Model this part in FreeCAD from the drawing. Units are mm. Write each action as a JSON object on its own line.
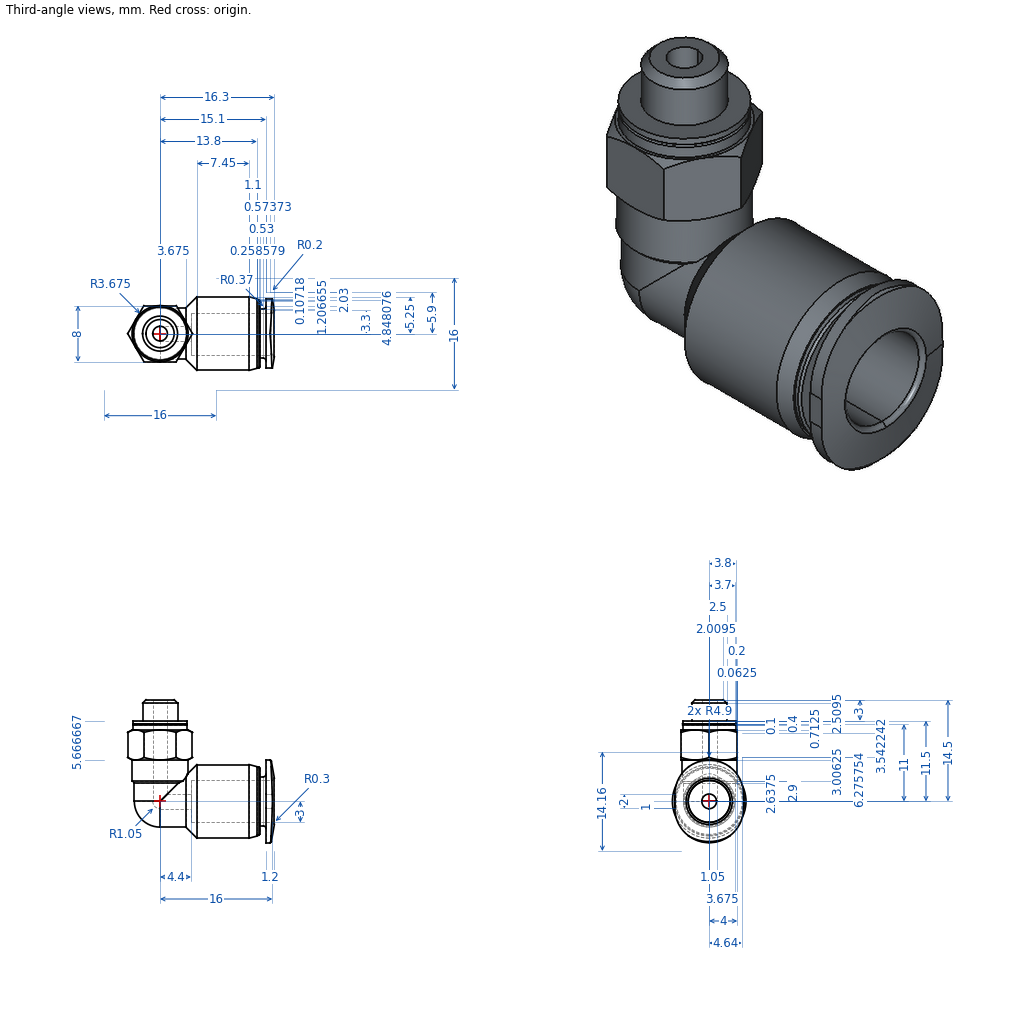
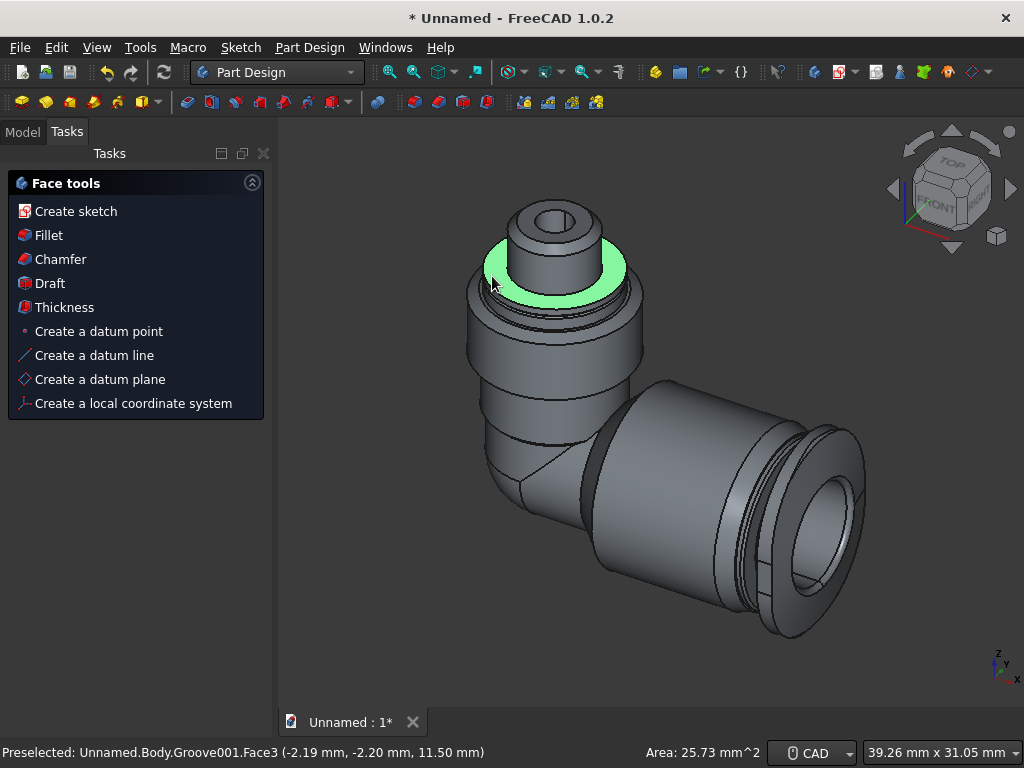
{"action": "left_click", "coordinate": [840, 72]}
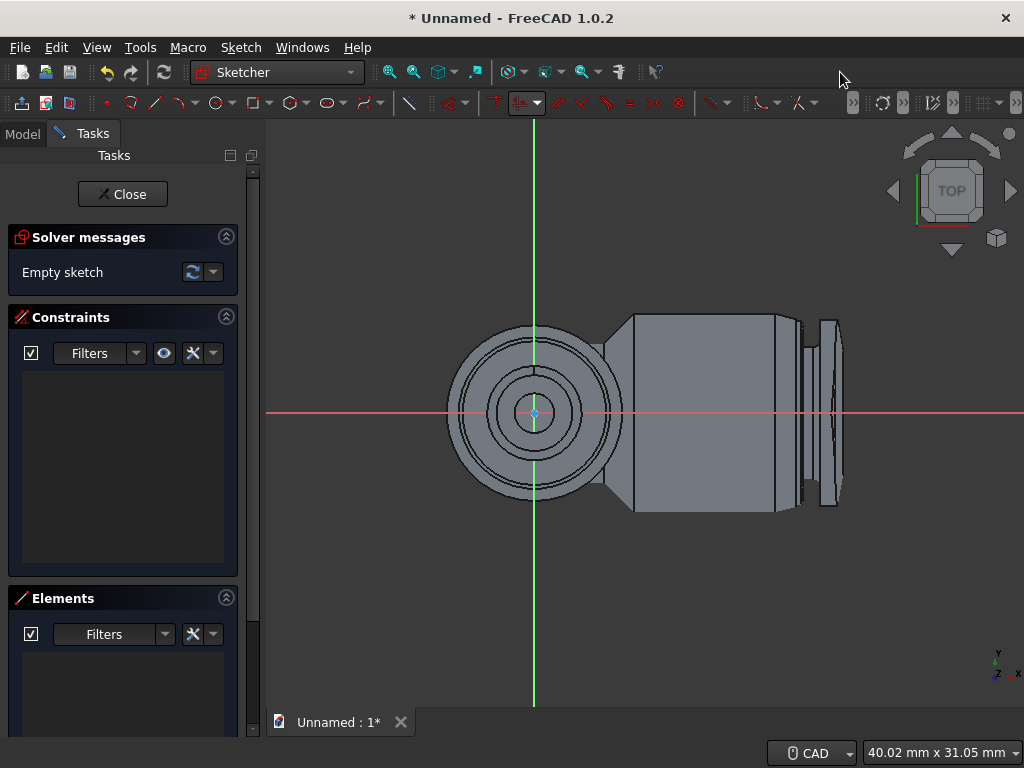
{"action": "left_click", "coordinate": [70, 104]}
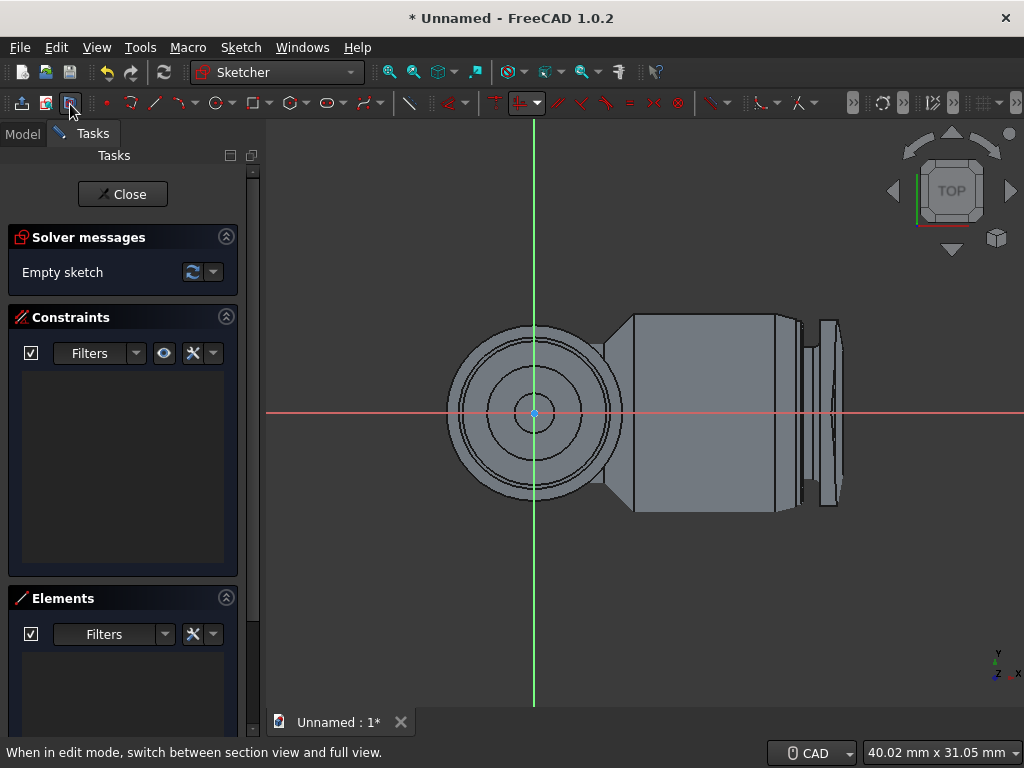
{"action": "key", "text": "g v"}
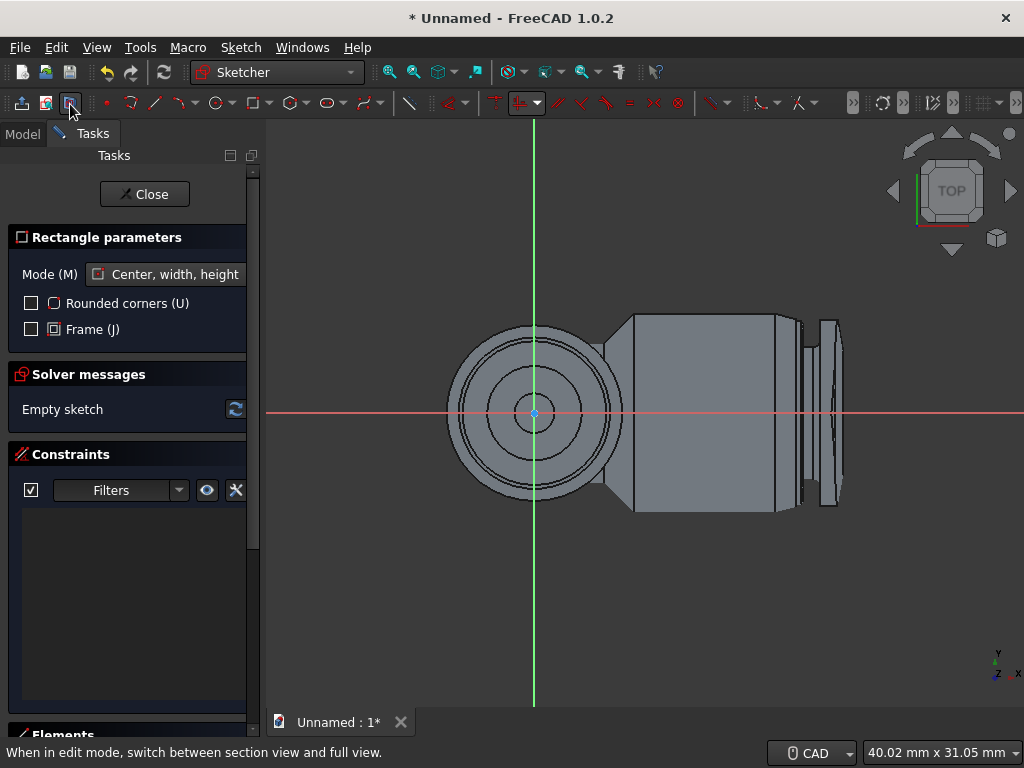
{"action": "left_click", "coordinate": [534, 413]}
{"action": "left_click", "coordinate": [686, 262]}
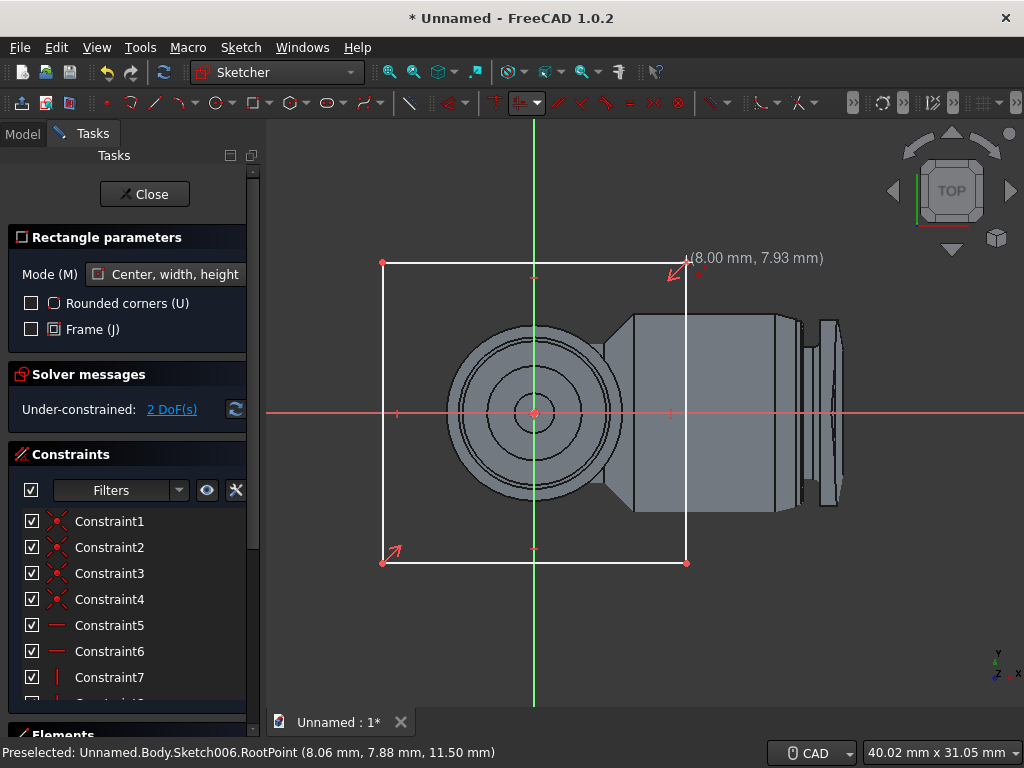
{"action": "left_click", "coordinate": [290, 104]}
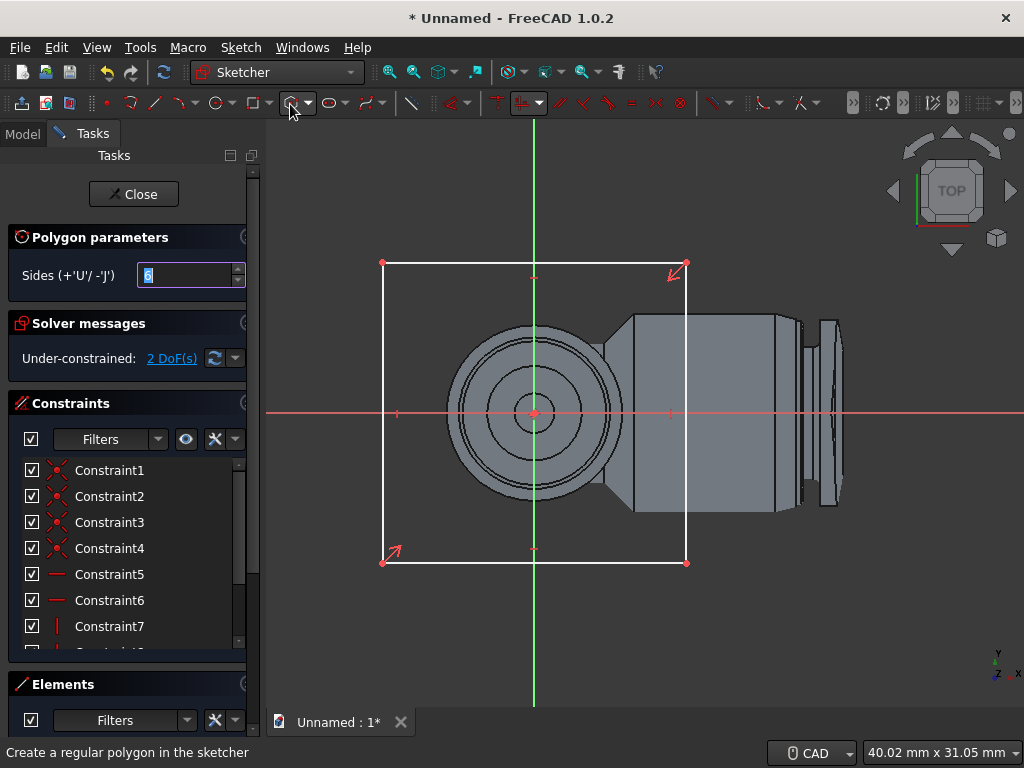
{"action": "left_click", "coordinate": [534, 413]}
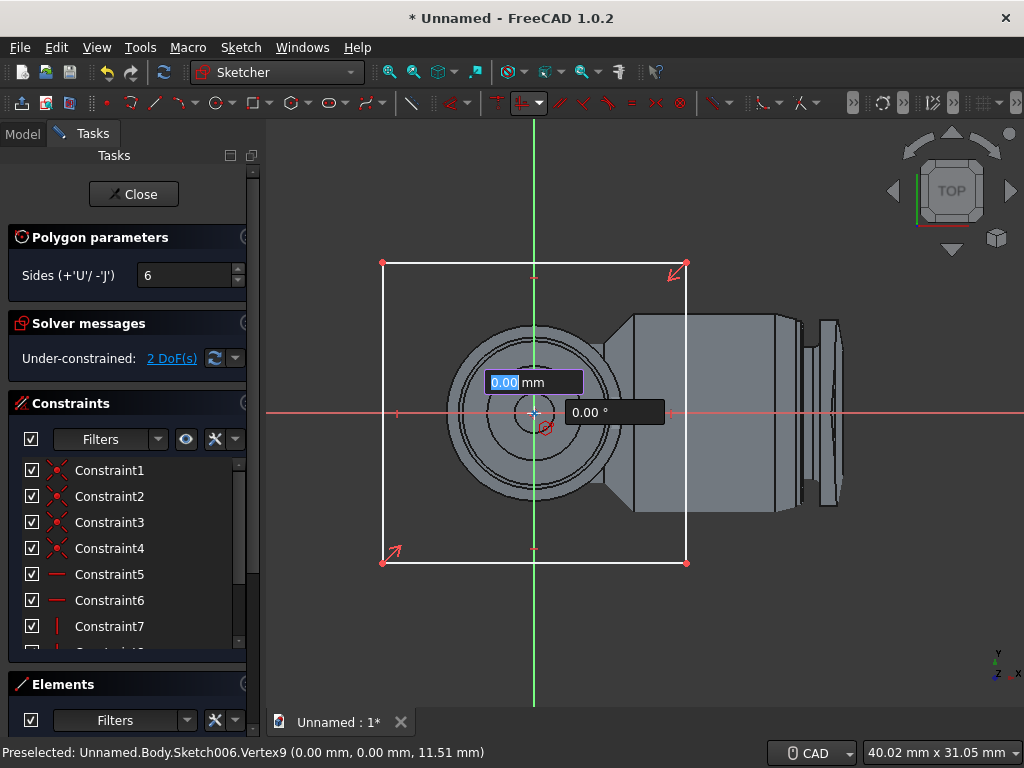
{"action": "left_click", "coordinate": [447, 413]}
{"action": "right_click", "coordinate": [447, 413]}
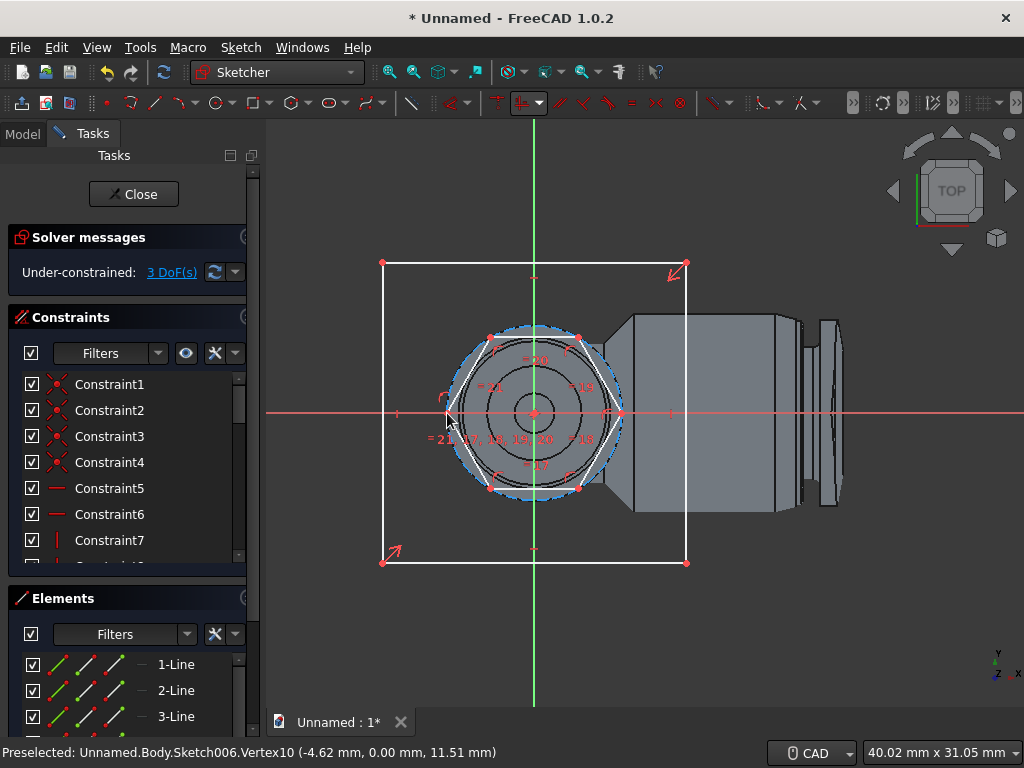
{"action": "left_click", "coordinate": [450, 104]}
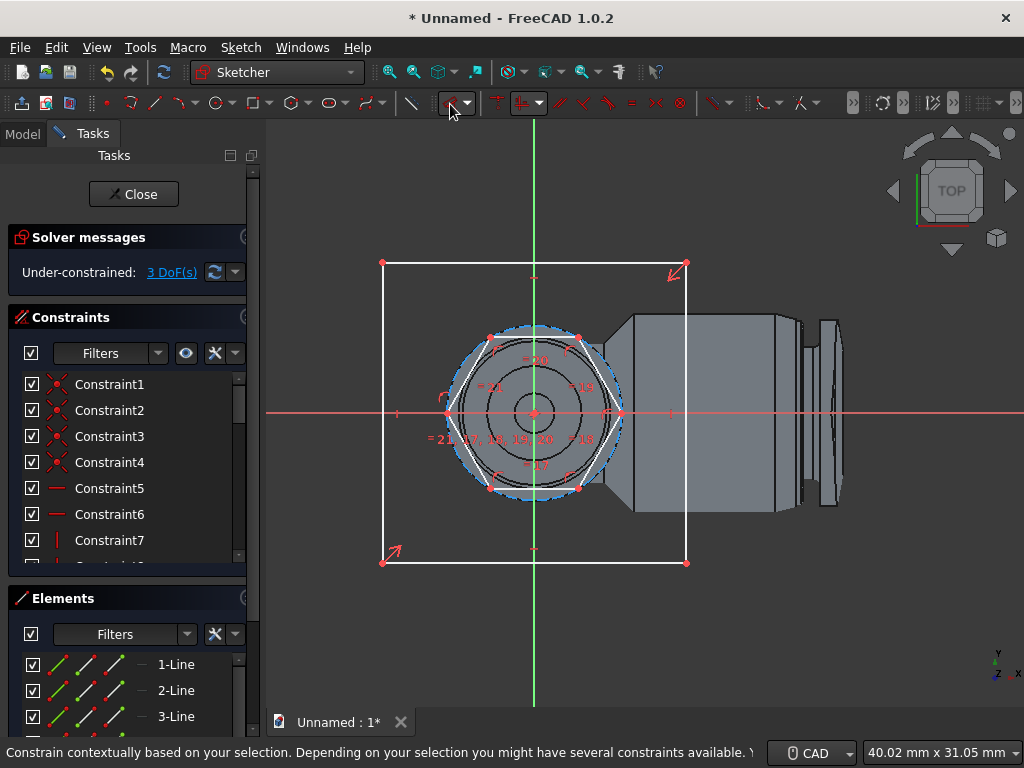
{"action": "left_click", "coordinate": [491, 489]}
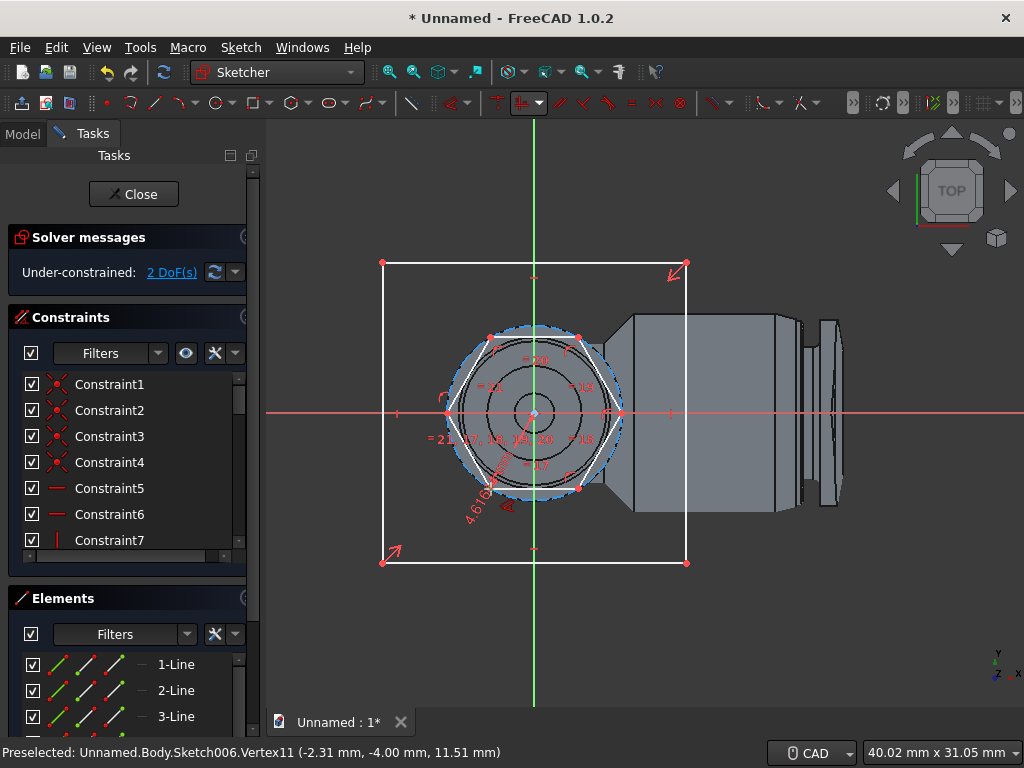
{"action": "left_click", "coordinate": [578, 337]}
{"action": "left_click", "coordinate": [636, 378]}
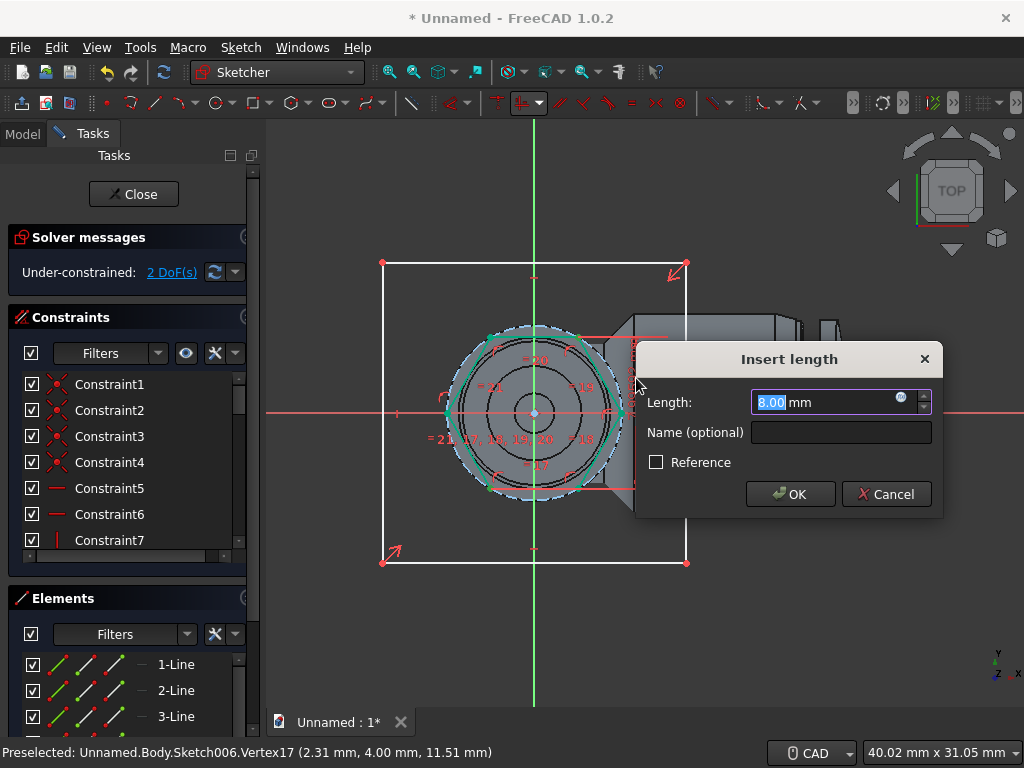
{"action": "type", "text": "8"}
{"action": "key", "text": "Return"}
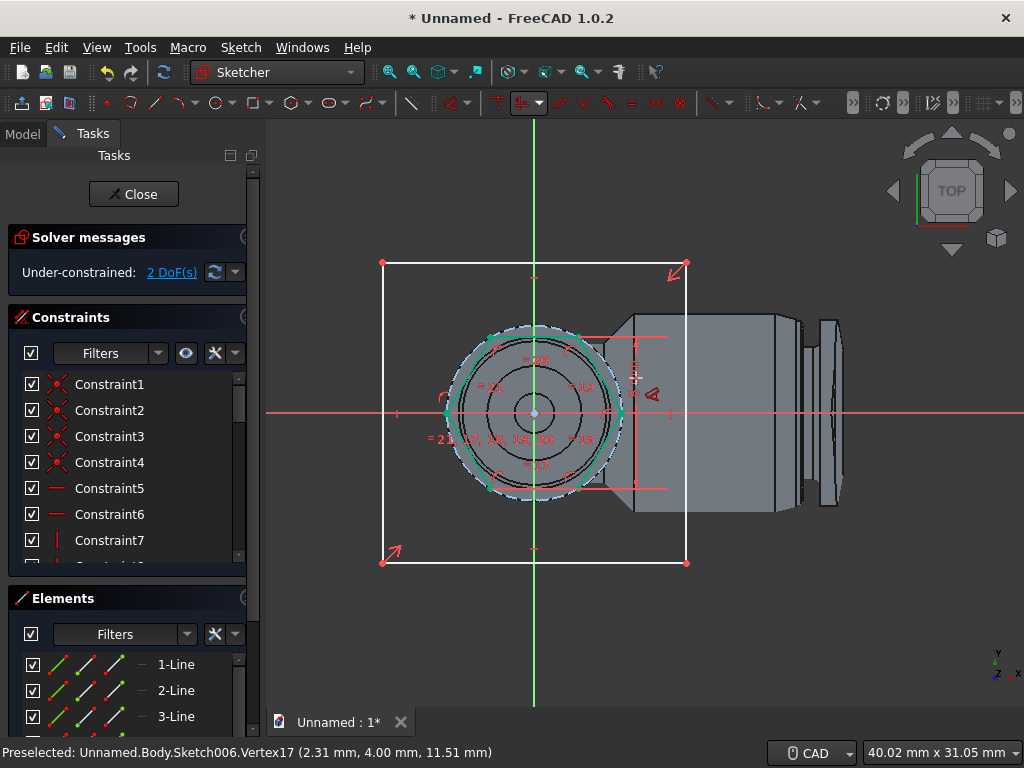
{"action": "left_click", "coordinate": [474, 563]}
{"action": "left_click", "coordinate": [465, 597]}